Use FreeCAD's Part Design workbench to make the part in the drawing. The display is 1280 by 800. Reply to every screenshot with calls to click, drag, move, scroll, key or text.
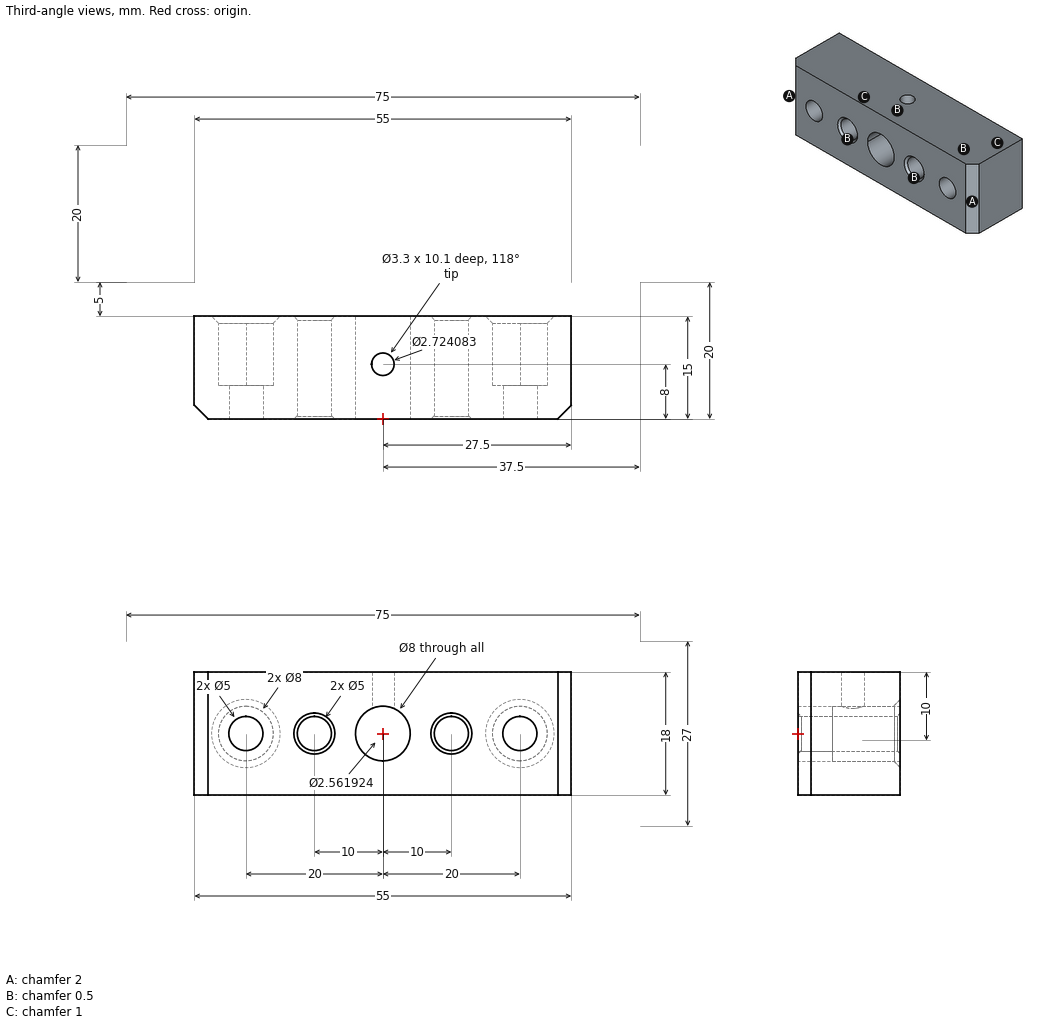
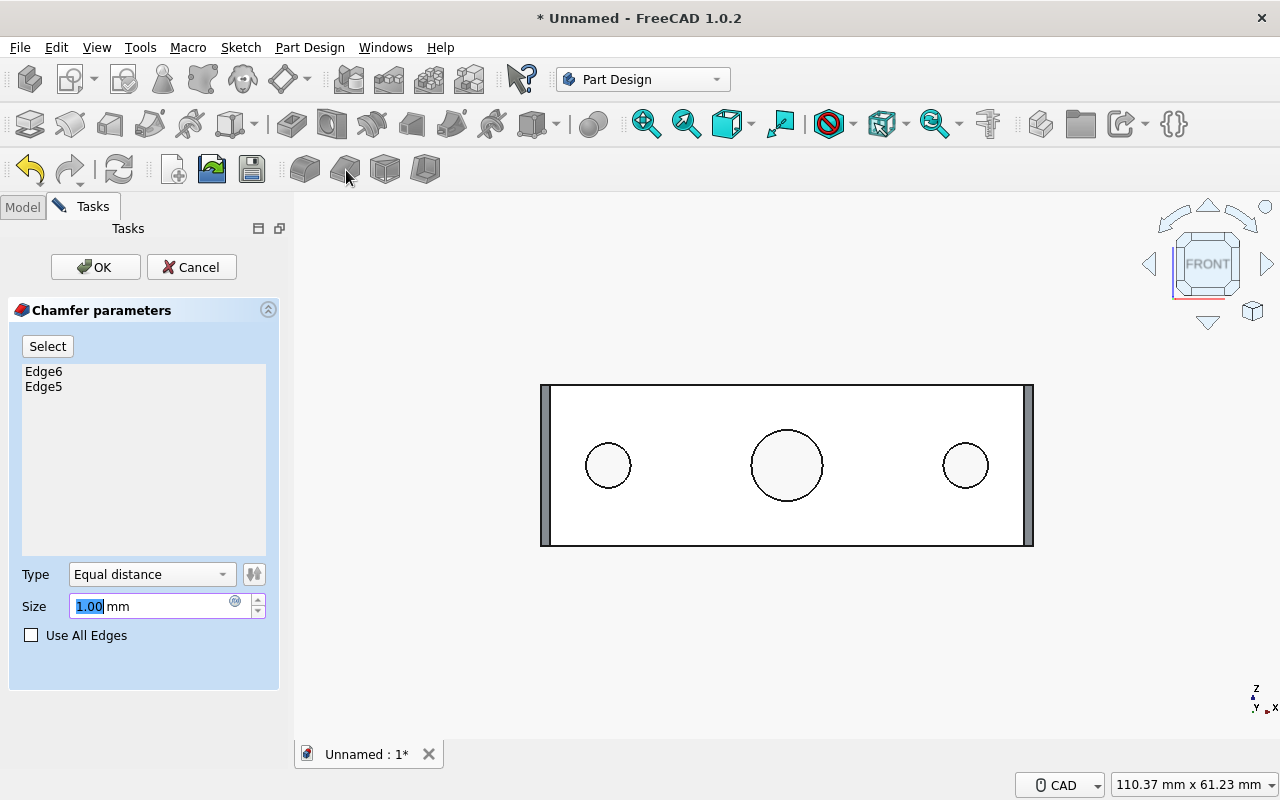
text(2)
key(Tab)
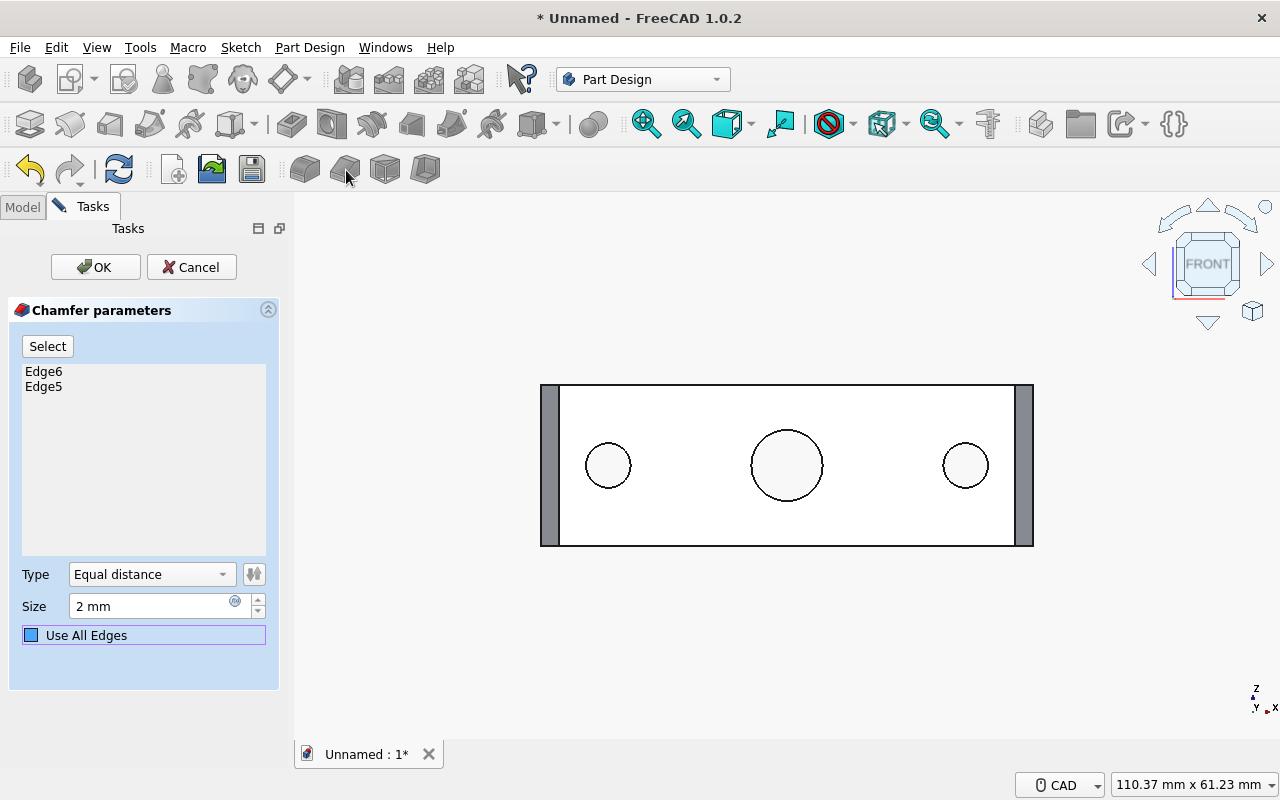
click(96, 267)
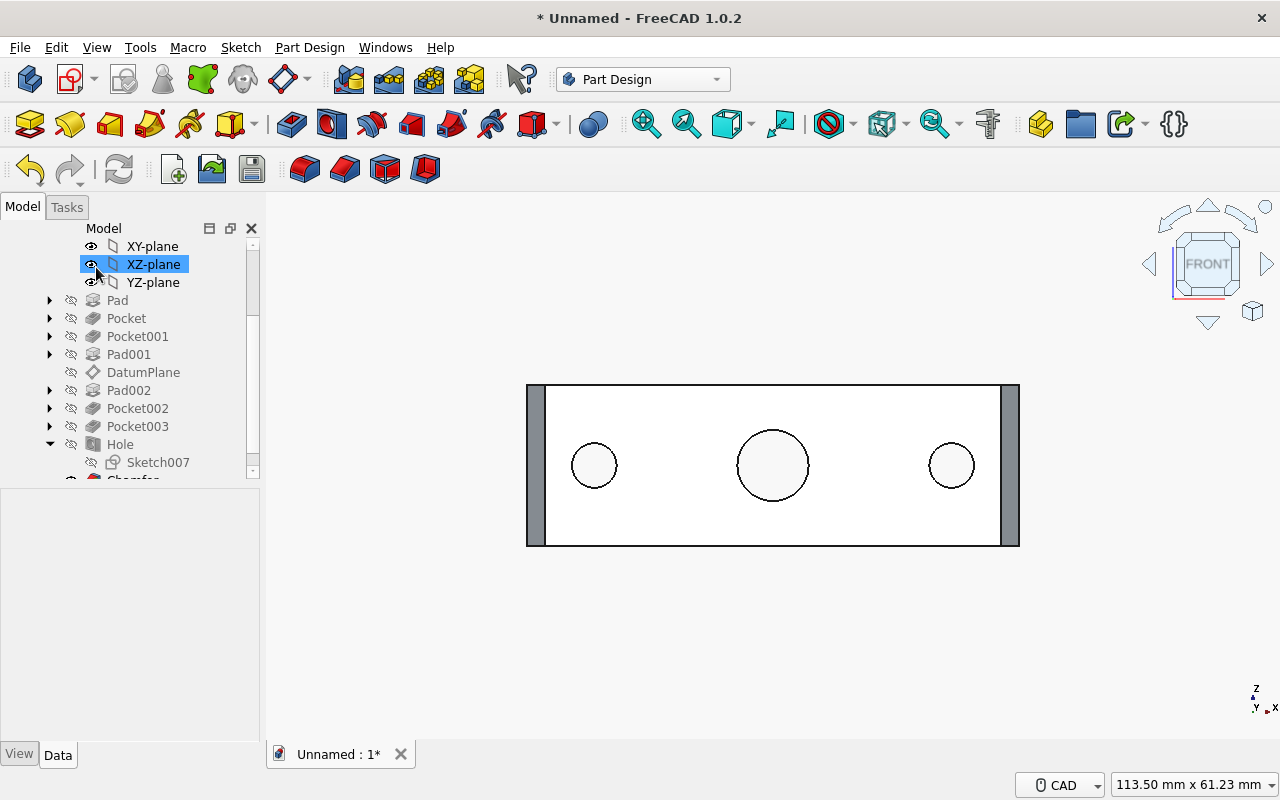
key(4)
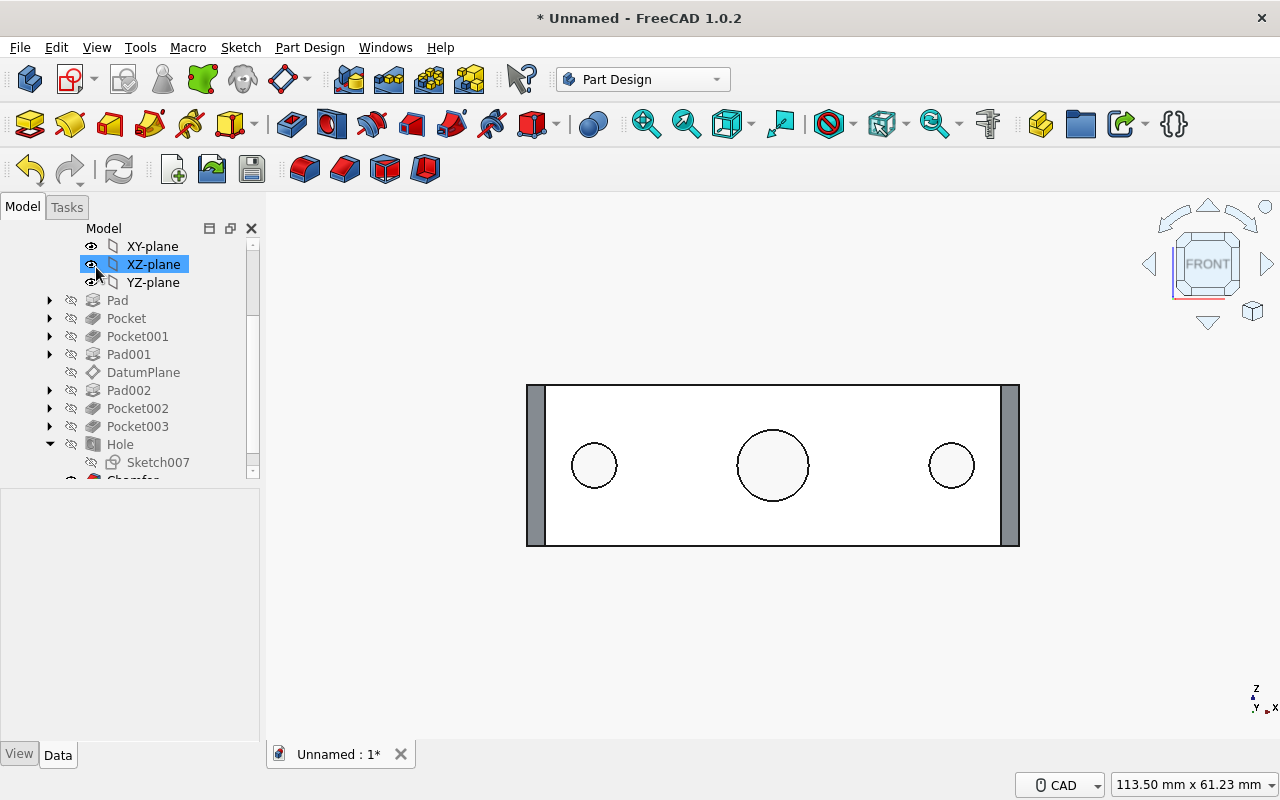
click(703, 487)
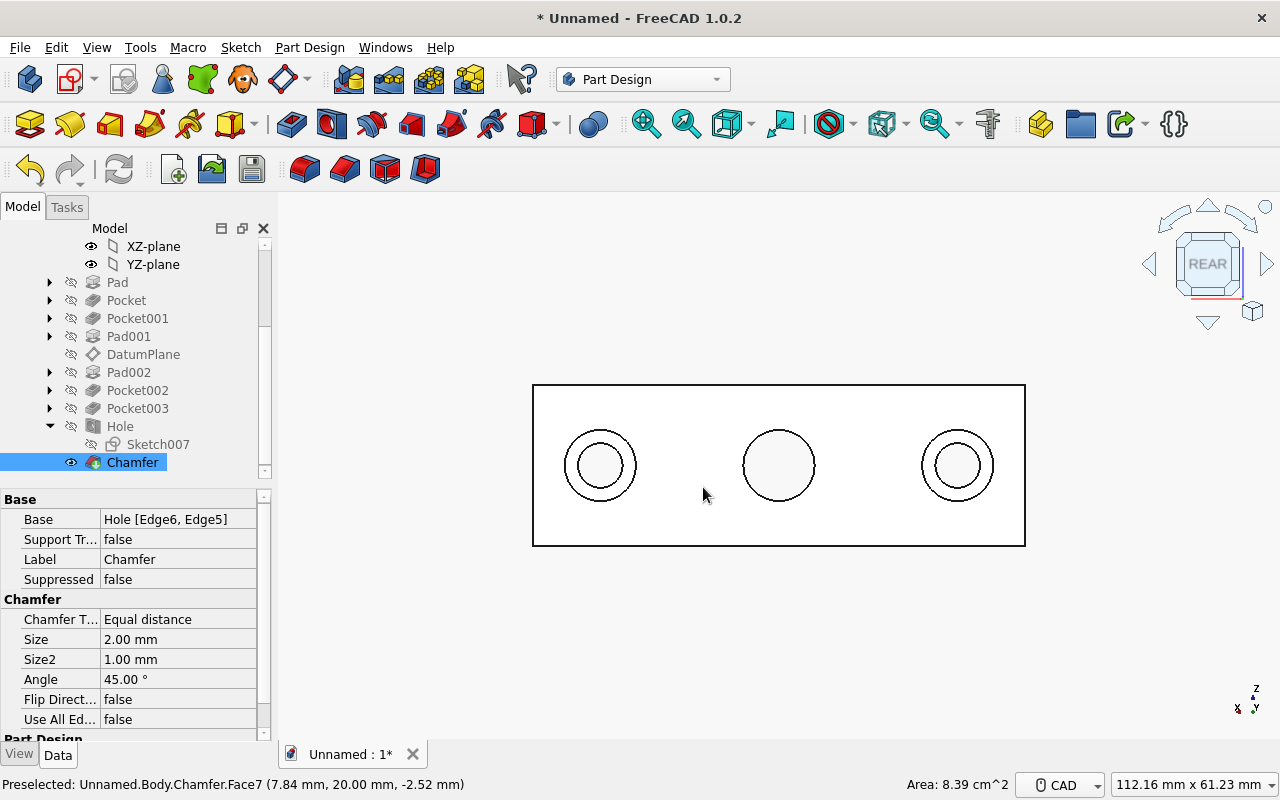
click(70, 80)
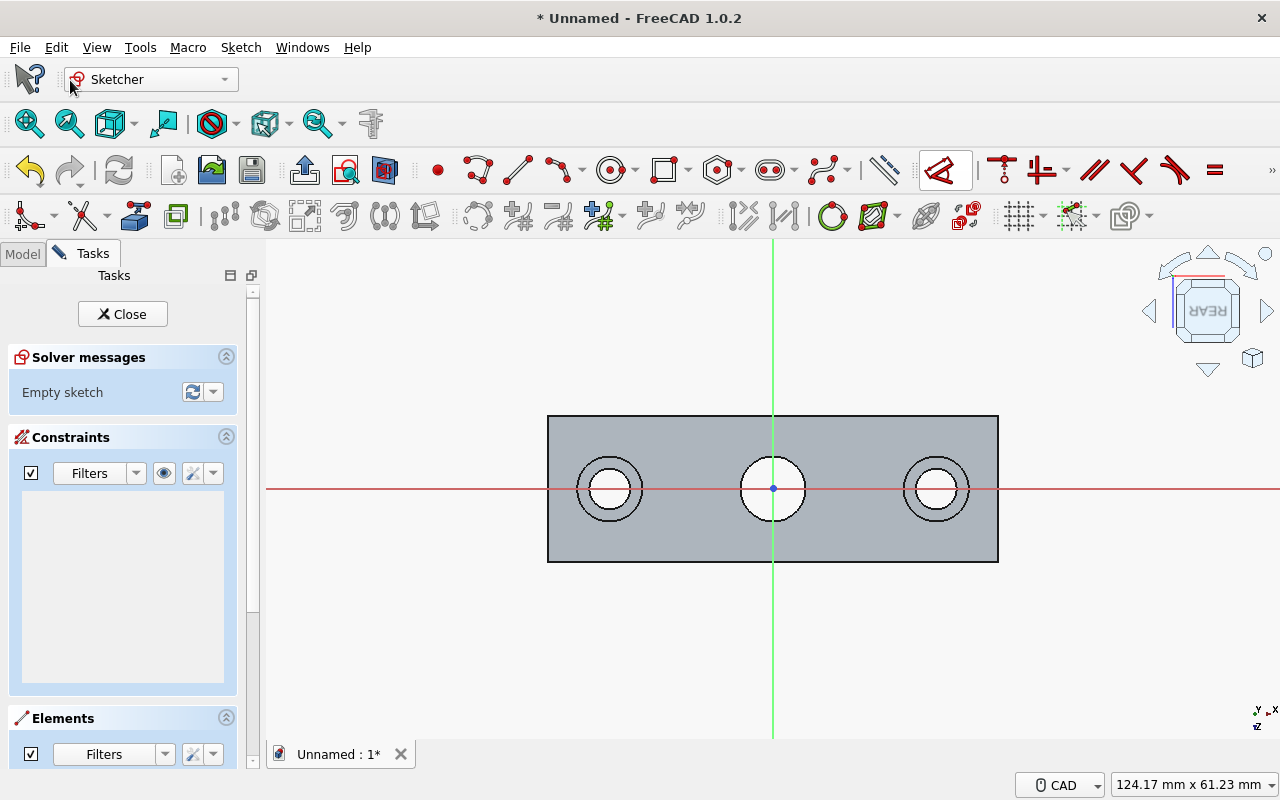
scroll(813, 489, up, 5)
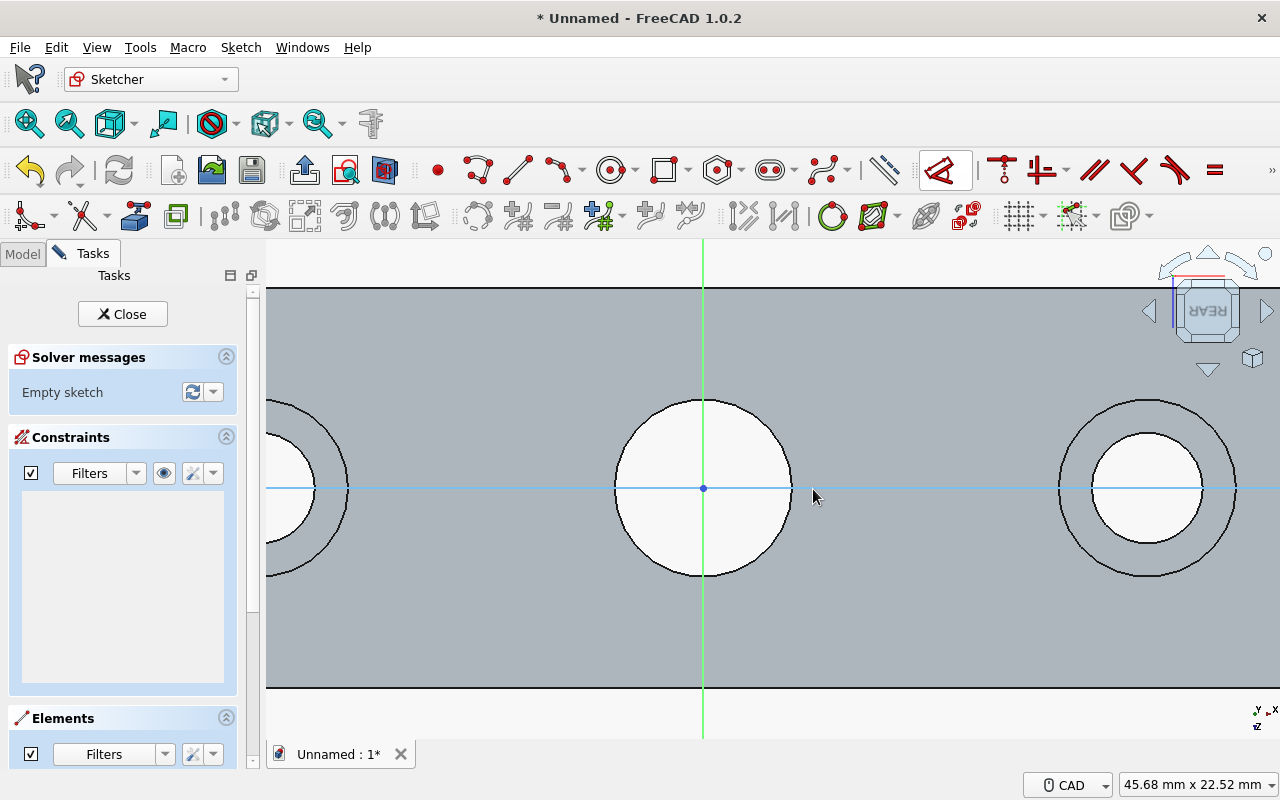
click(612, 170)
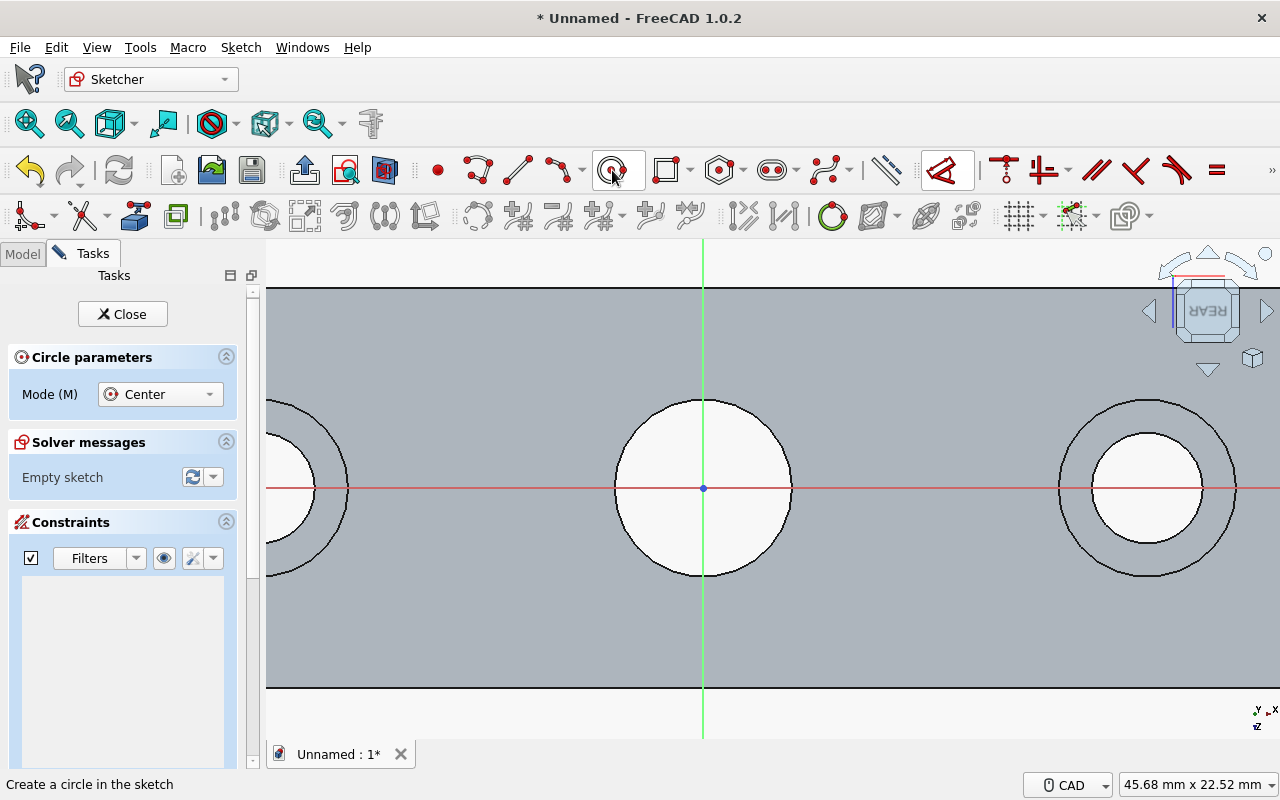
click(481, 488)
move(521, 449)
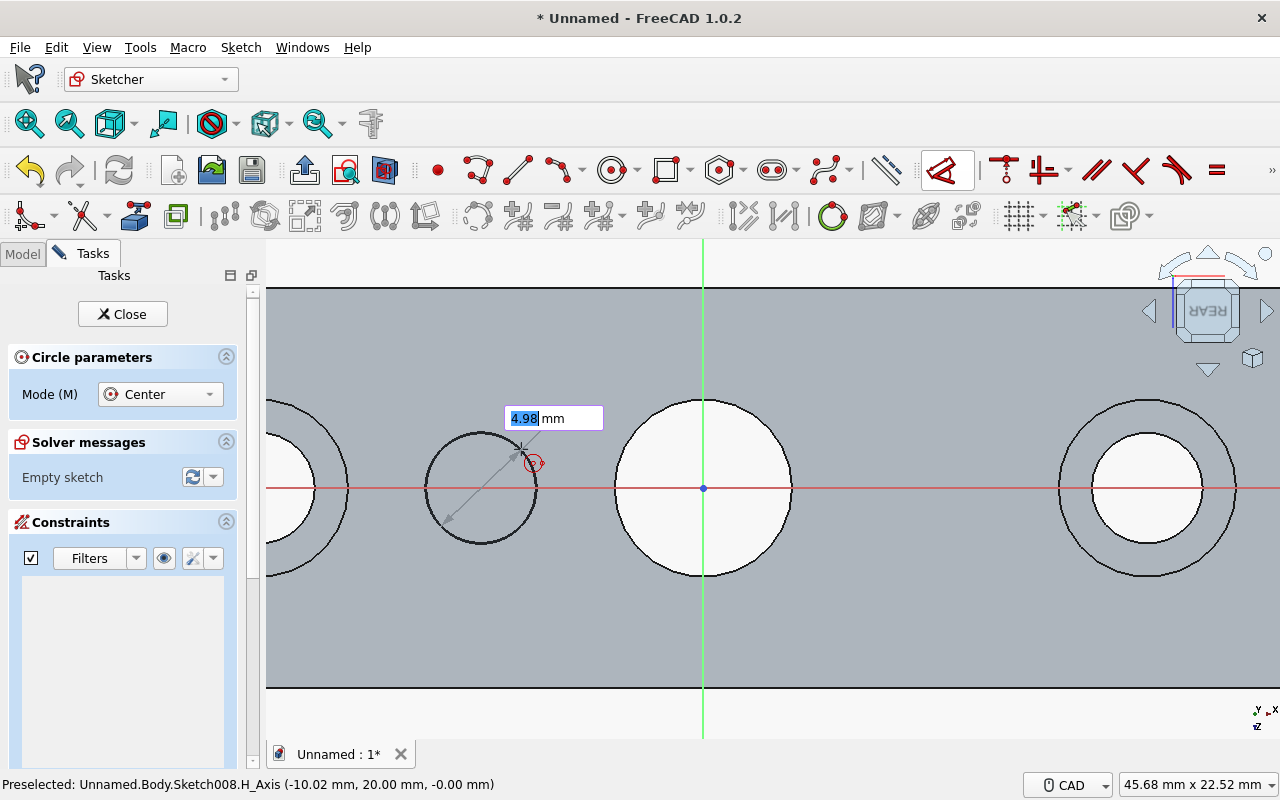
text(5)
key(Return)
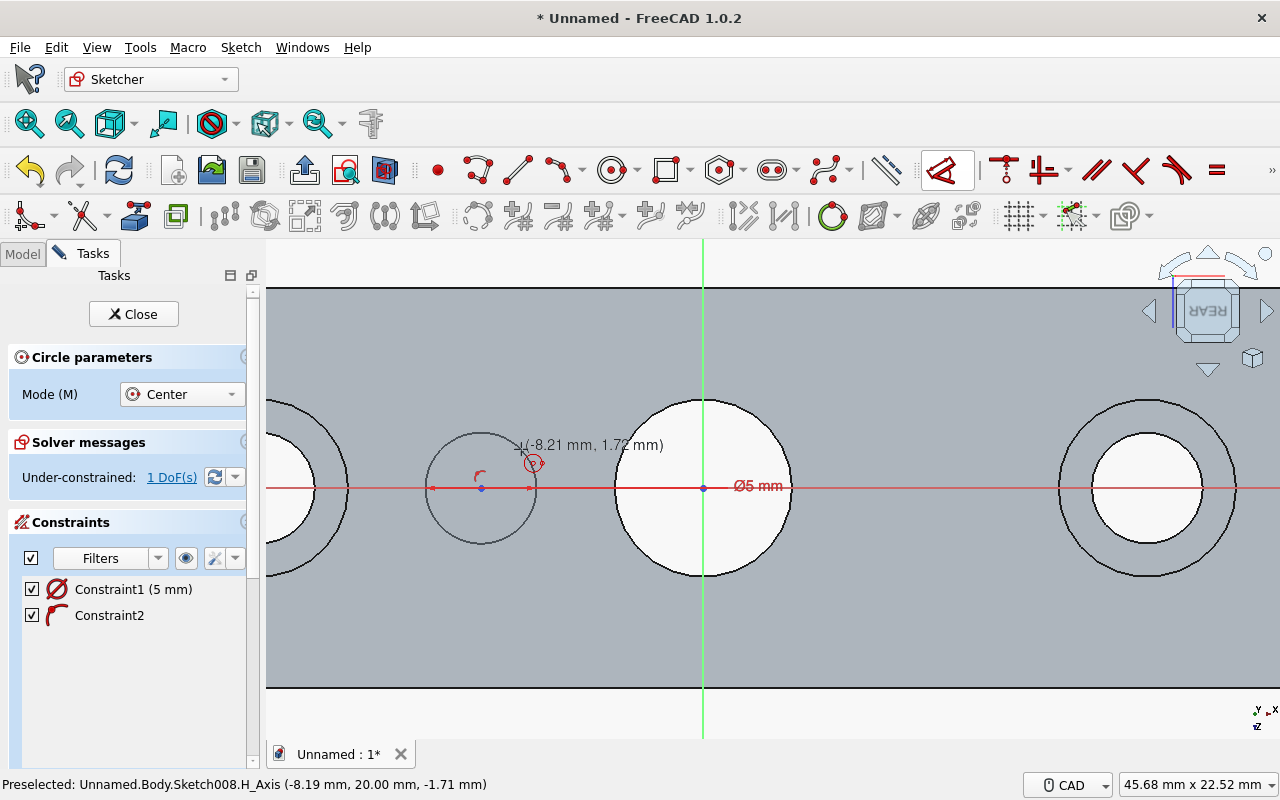
click(925, 488)
move(965, 449)